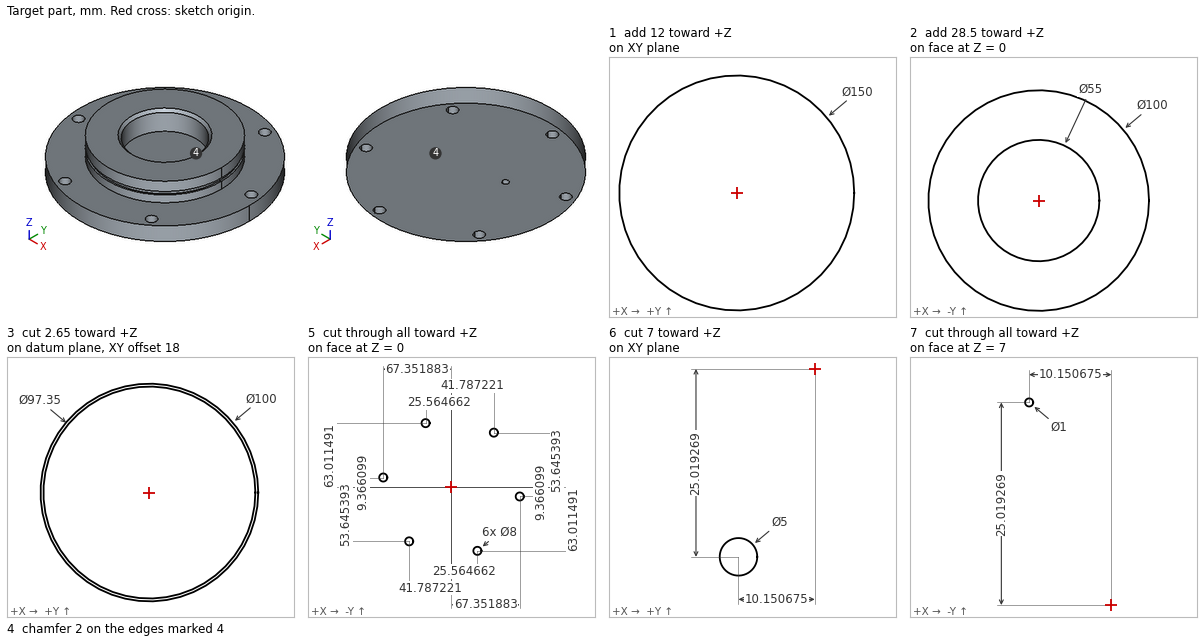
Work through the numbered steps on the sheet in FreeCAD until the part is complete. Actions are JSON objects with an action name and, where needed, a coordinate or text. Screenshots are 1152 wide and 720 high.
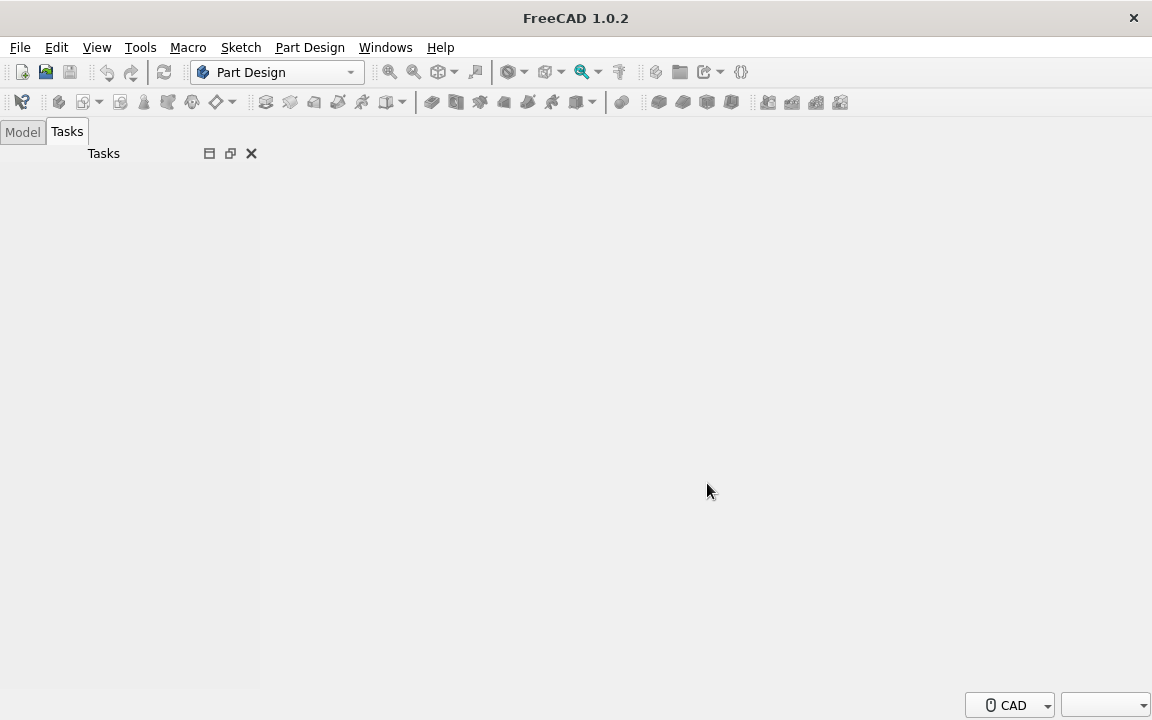
{"action": "key", "text": "ctrl+n"}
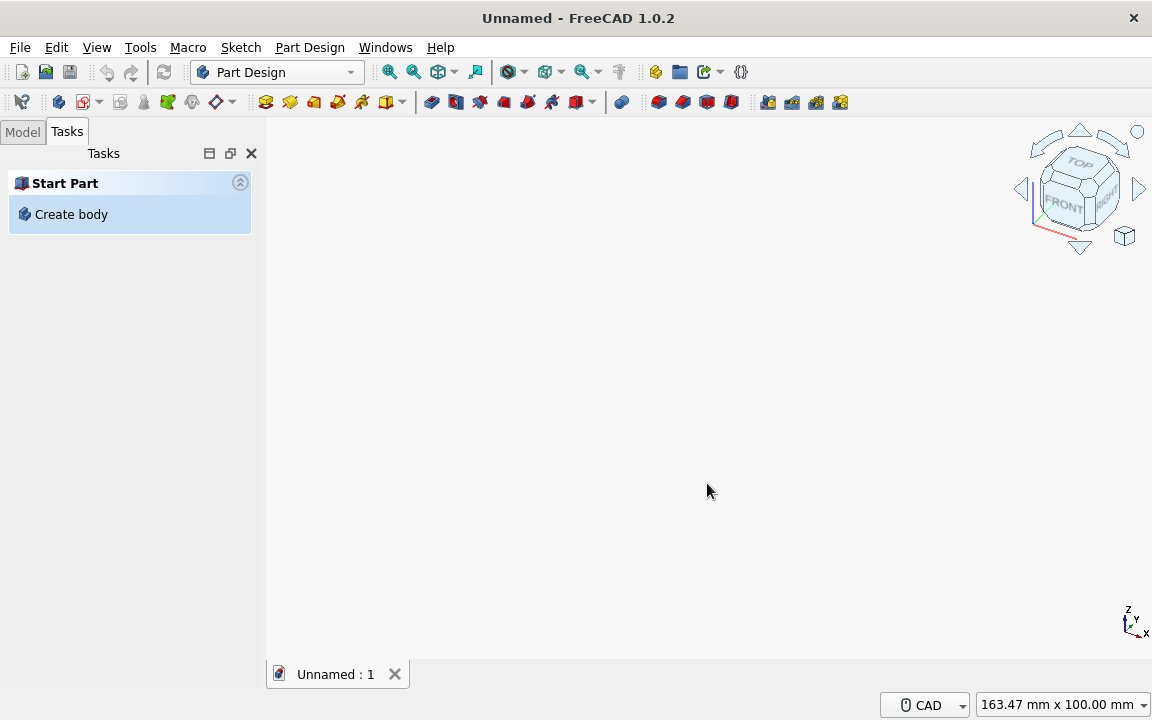
{"action": "left_click", "coordinate": [84, 102]}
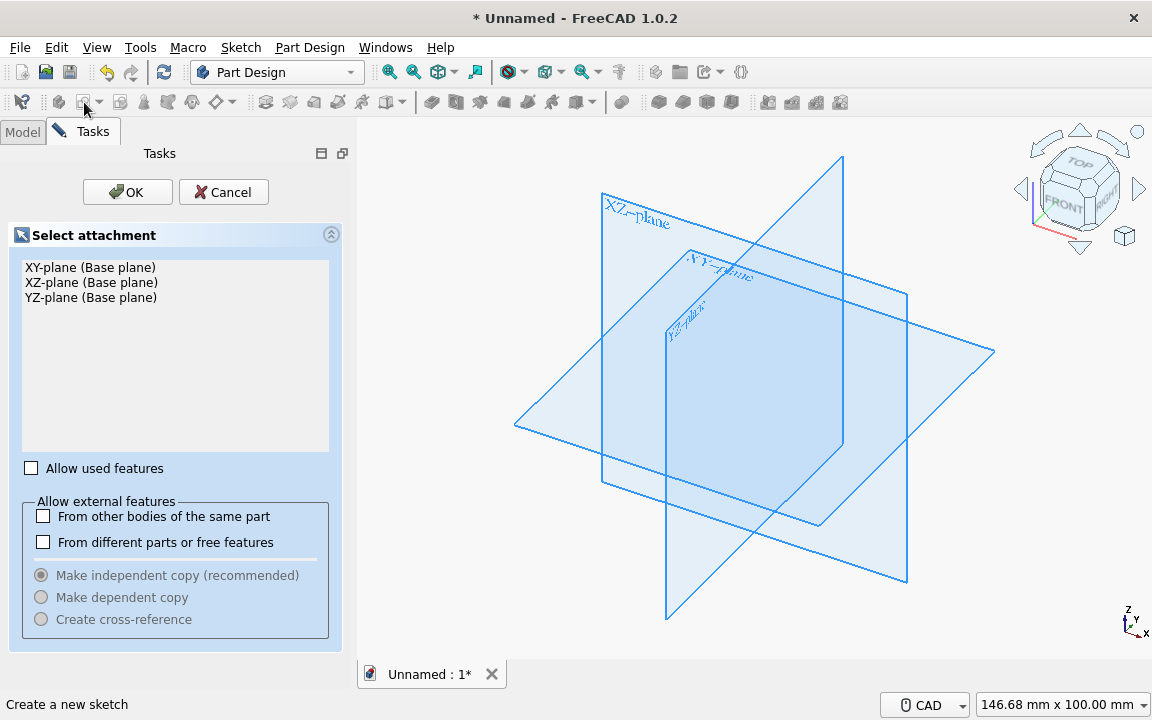
{"action": "left_click", "coordinate": [82, 268]}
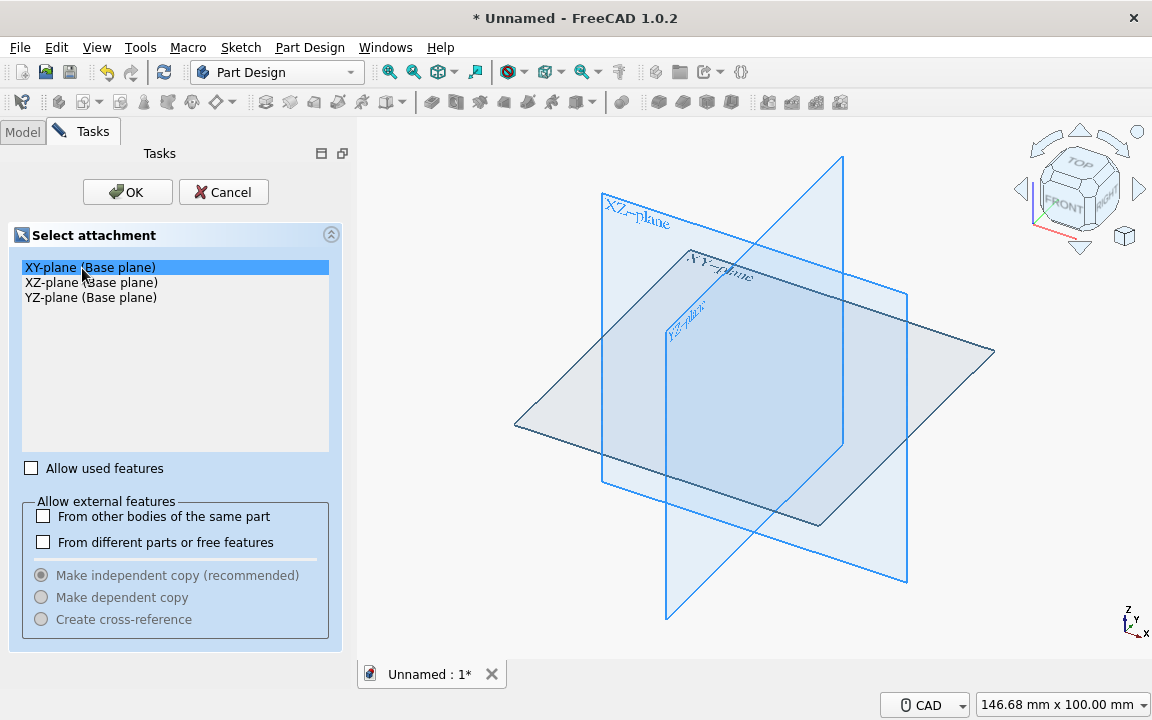
{"action": "left_click", "coordinate": [128, 192]}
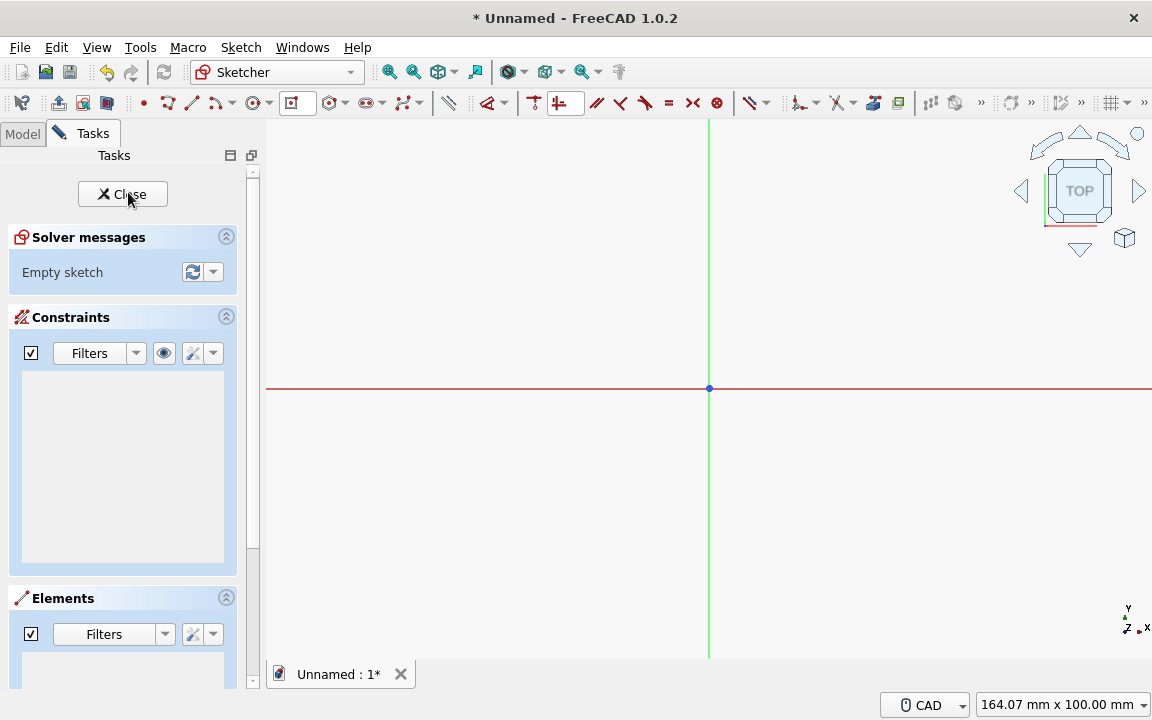
{"action": "scroll", "coordinate": [585, 389], "scroll_direction": "down", "scroll_amount": 4}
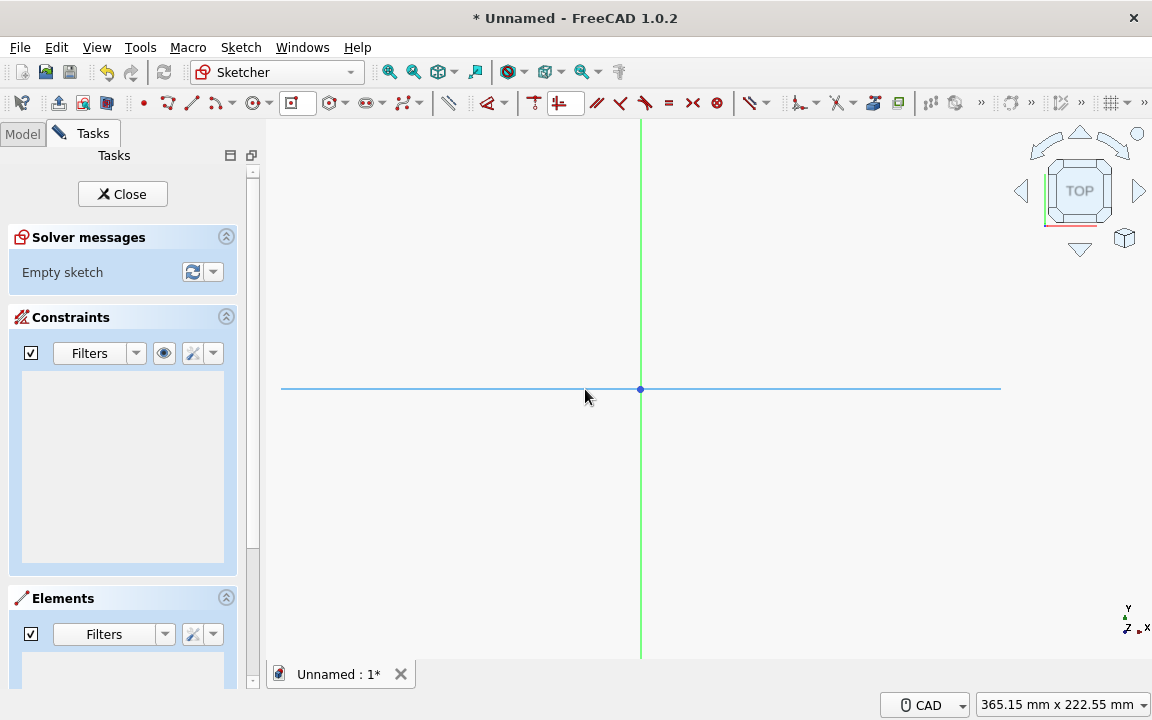
{"action": "left_click", "coordinate": [254, 104]}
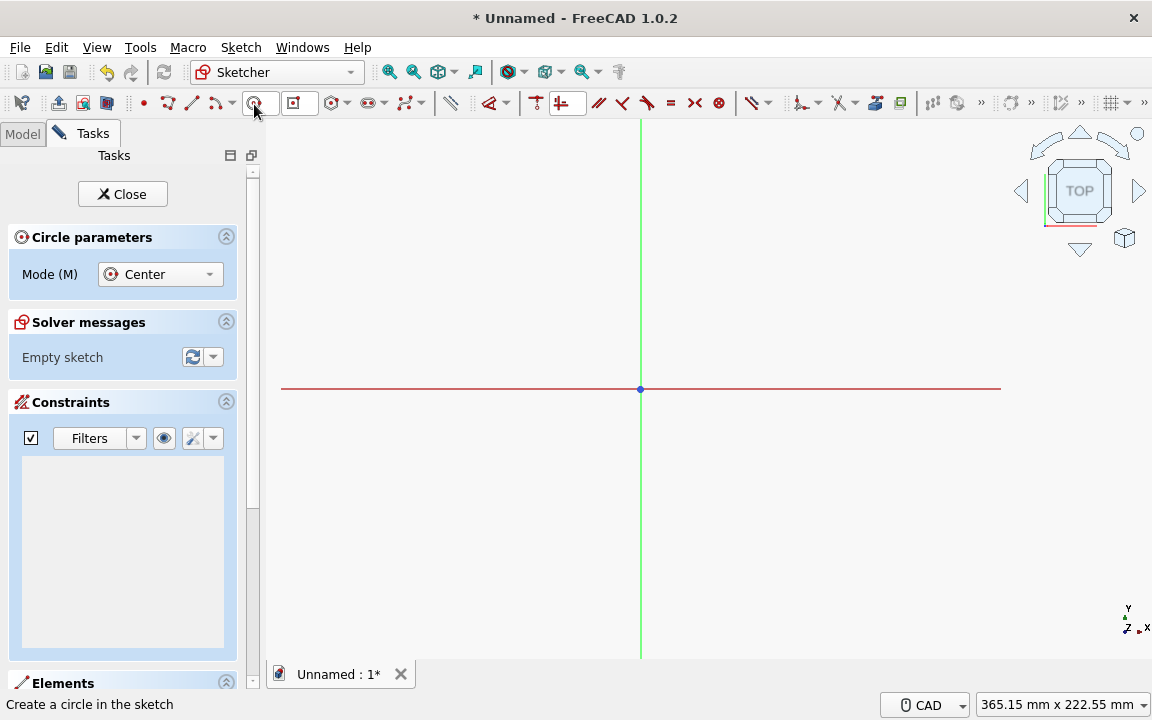
{"action": "left_click", "coordinate": [641, 389]}
{"action": "mouse_move", "coordinate": [770, 261]}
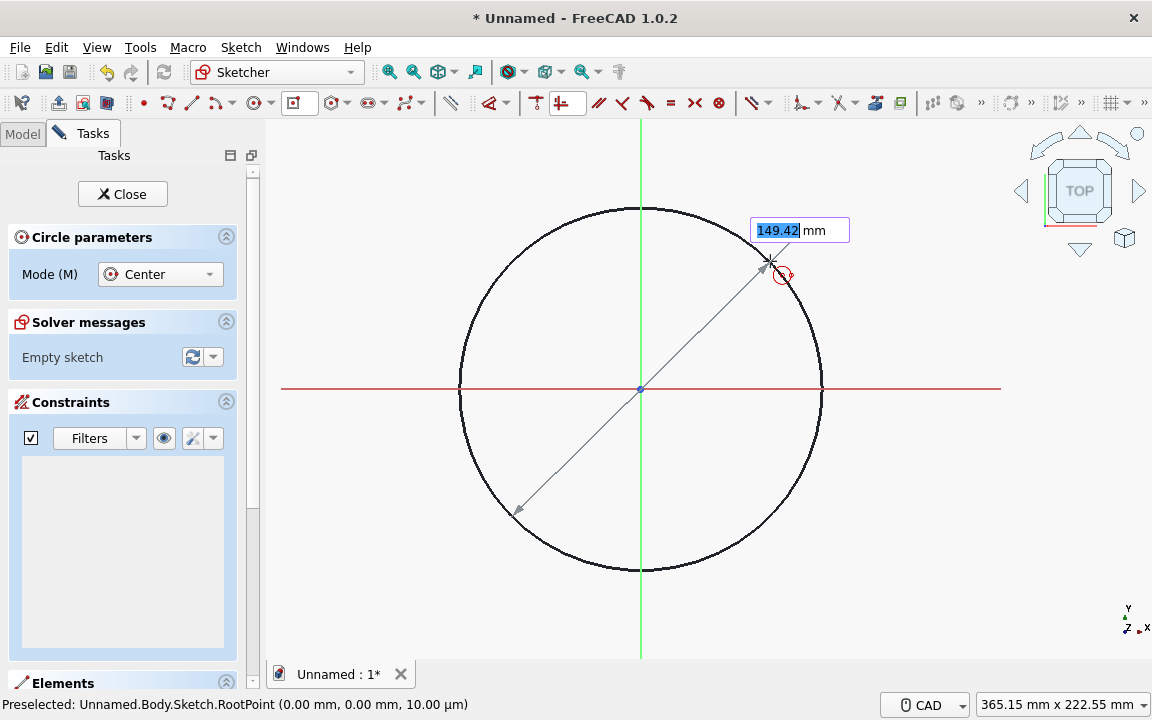
{"action": "type", "text": "150"}
{"action": "key", "text": "Return"}
{"action": "key", "text": "Escape"}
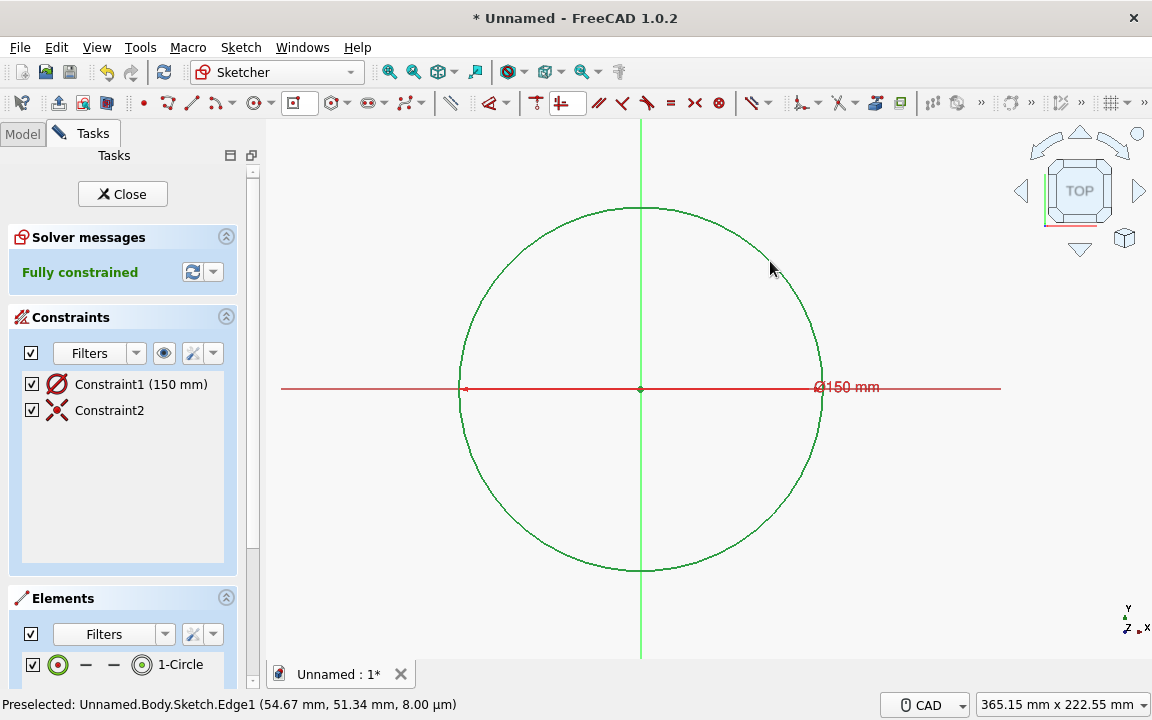
{"action": "left_click", "coordinate": [123, 194]}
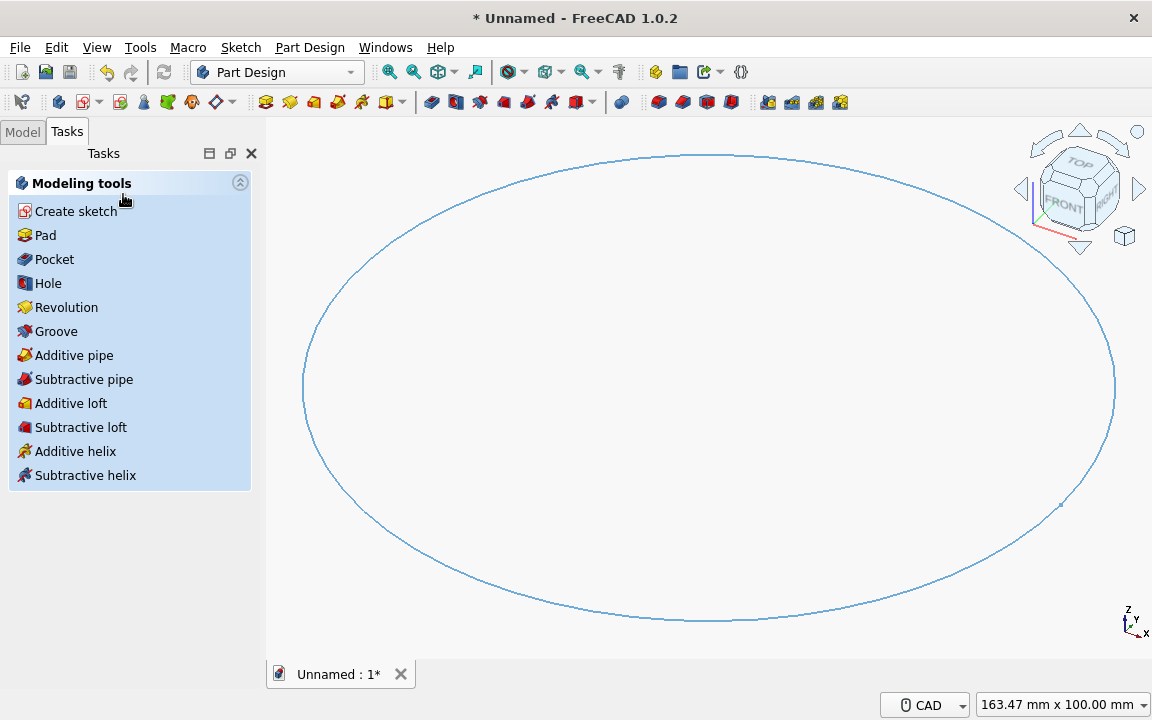
{"action": "left_click", "coordinate": [266, 102]}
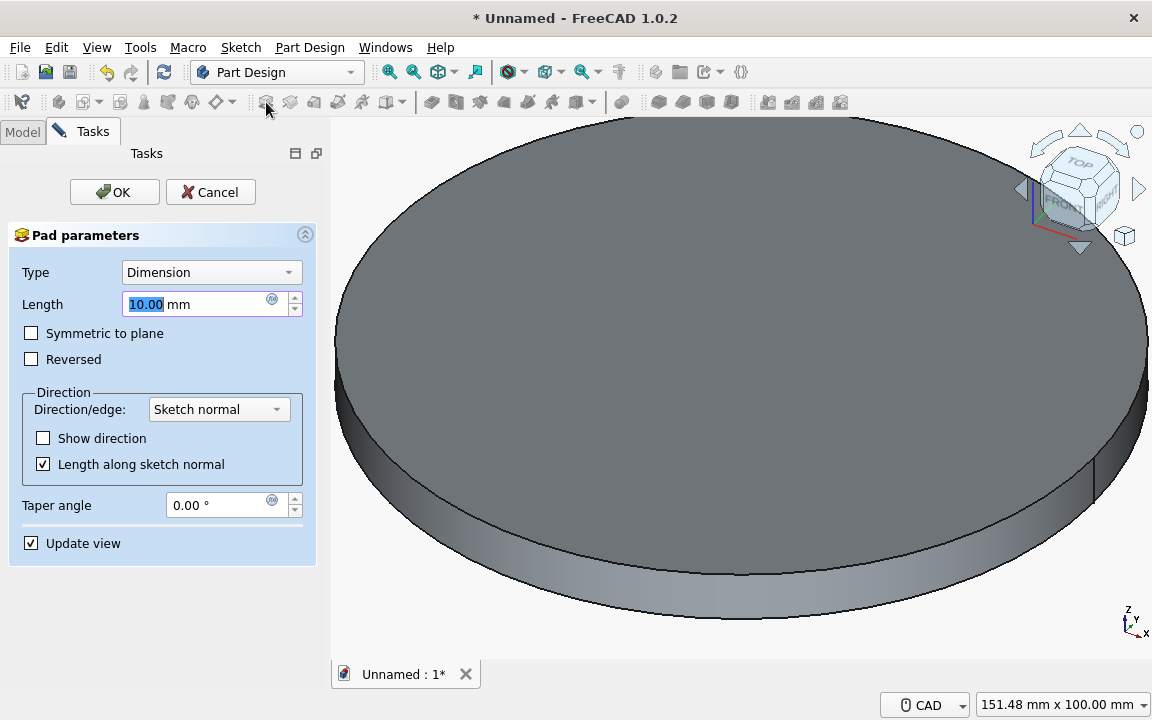
{"action": "type", "text": "12"}
{"action": "key", "text": "Tab"}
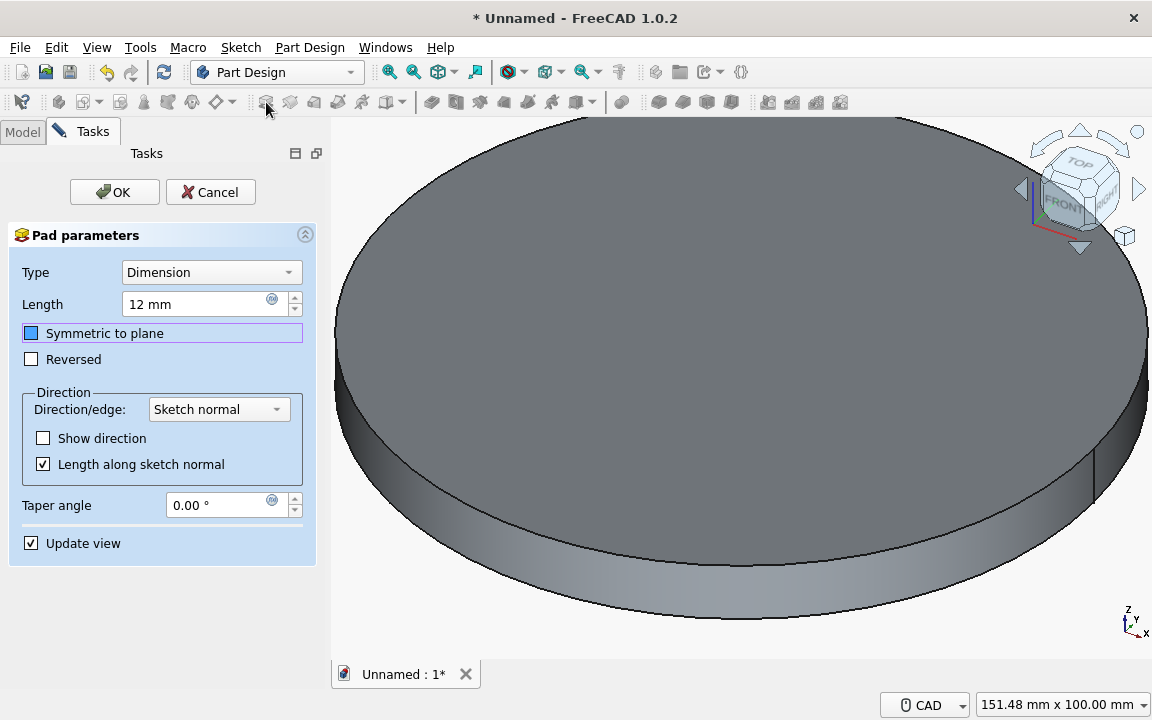
{"action": "left_click", "coordinate": [115, 192]}